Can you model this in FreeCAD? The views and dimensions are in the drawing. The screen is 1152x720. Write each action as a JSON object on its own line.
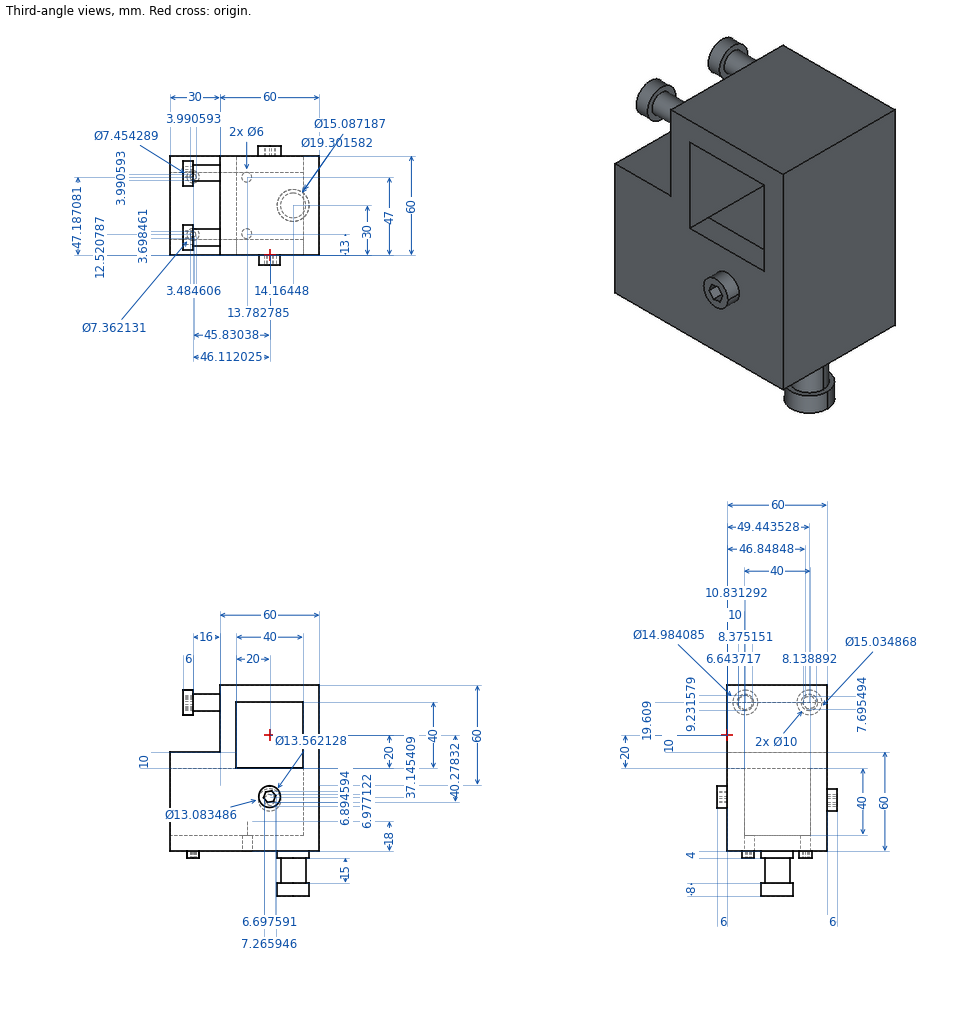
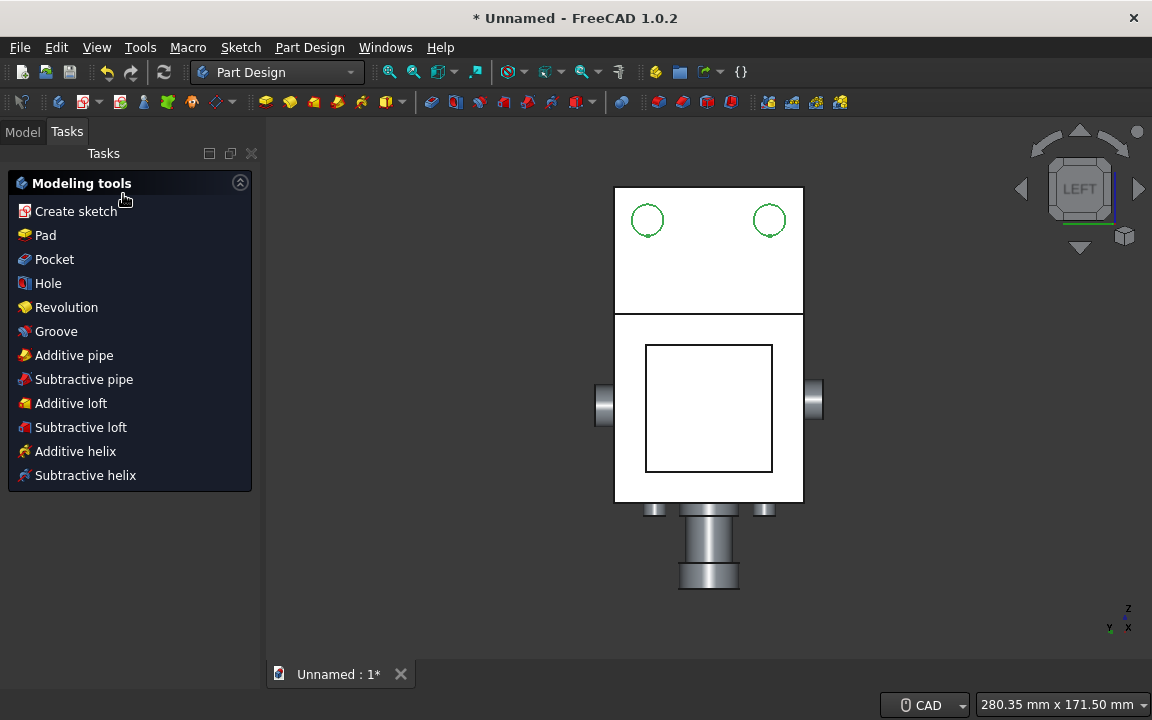
{"action": "left_click", "coordinate": [266, 102]}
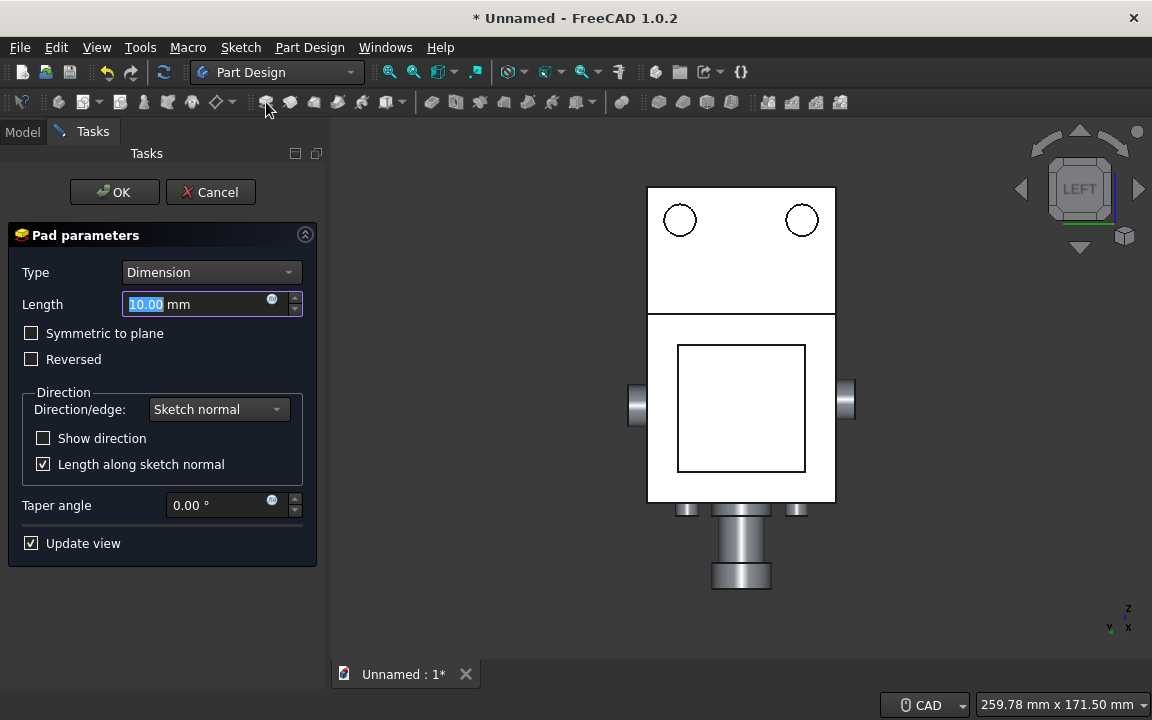
{"action": "type", "text": "16"}
{"action": "key", "text": "Tab"}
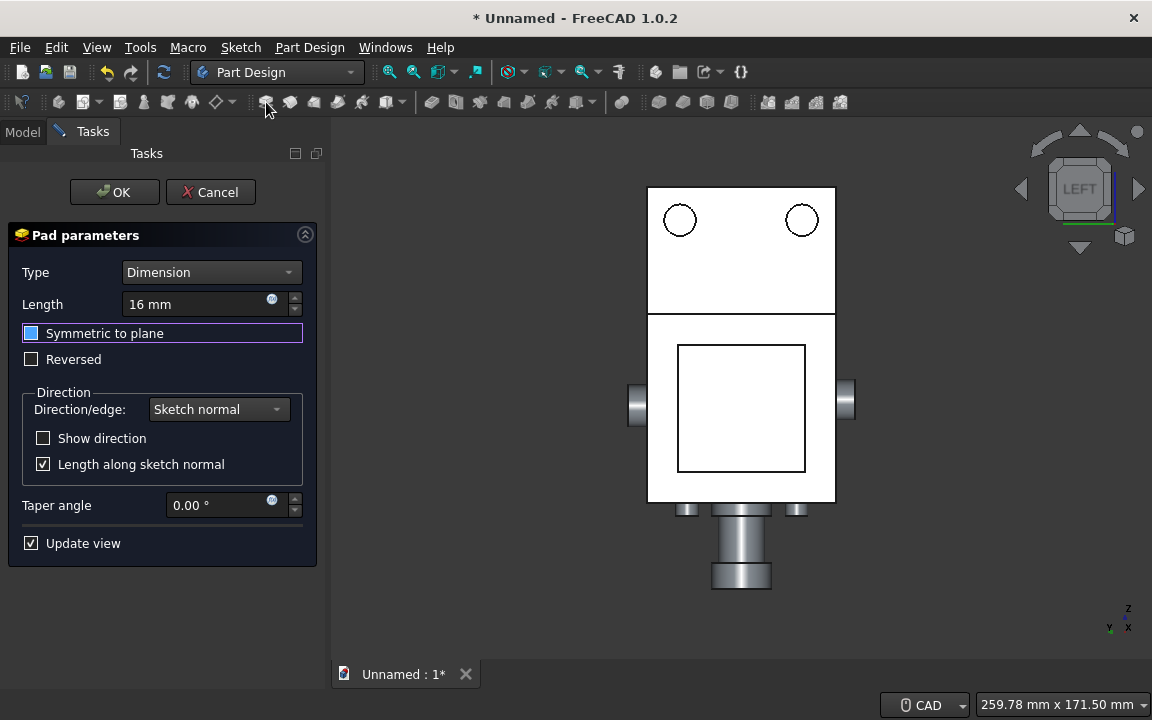
{"action": "left_click", "coordinate": [115, 192]}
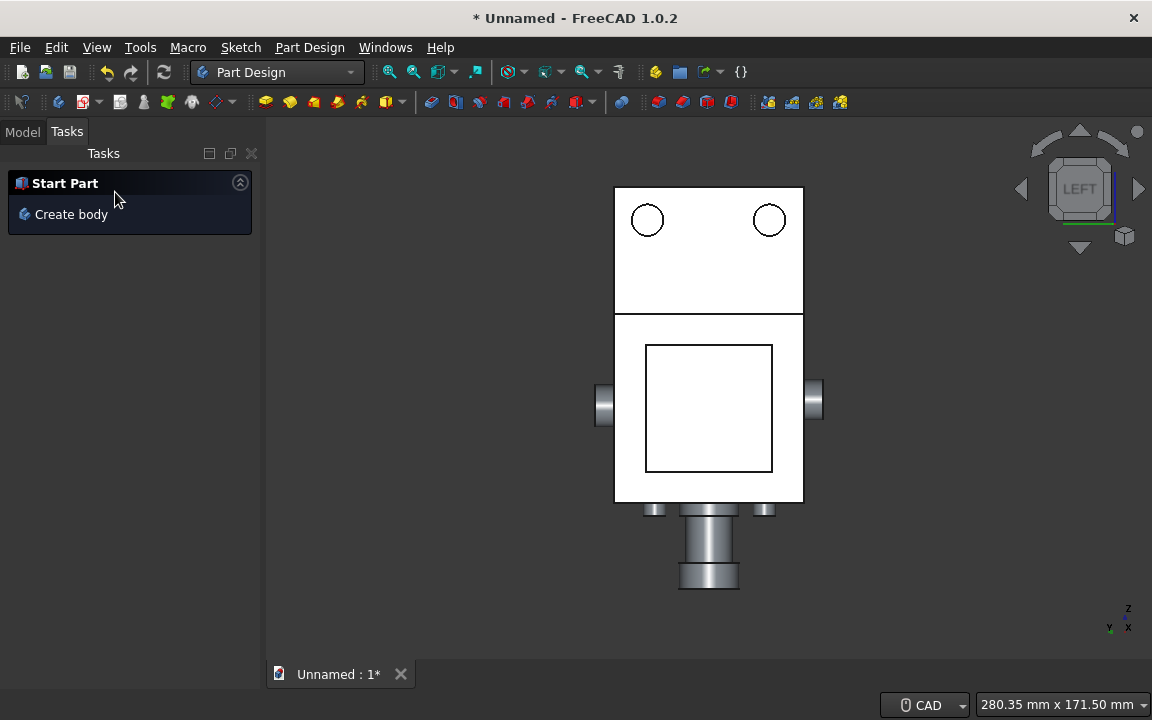
{"action": "left_click", "coordinate": [770, 219]}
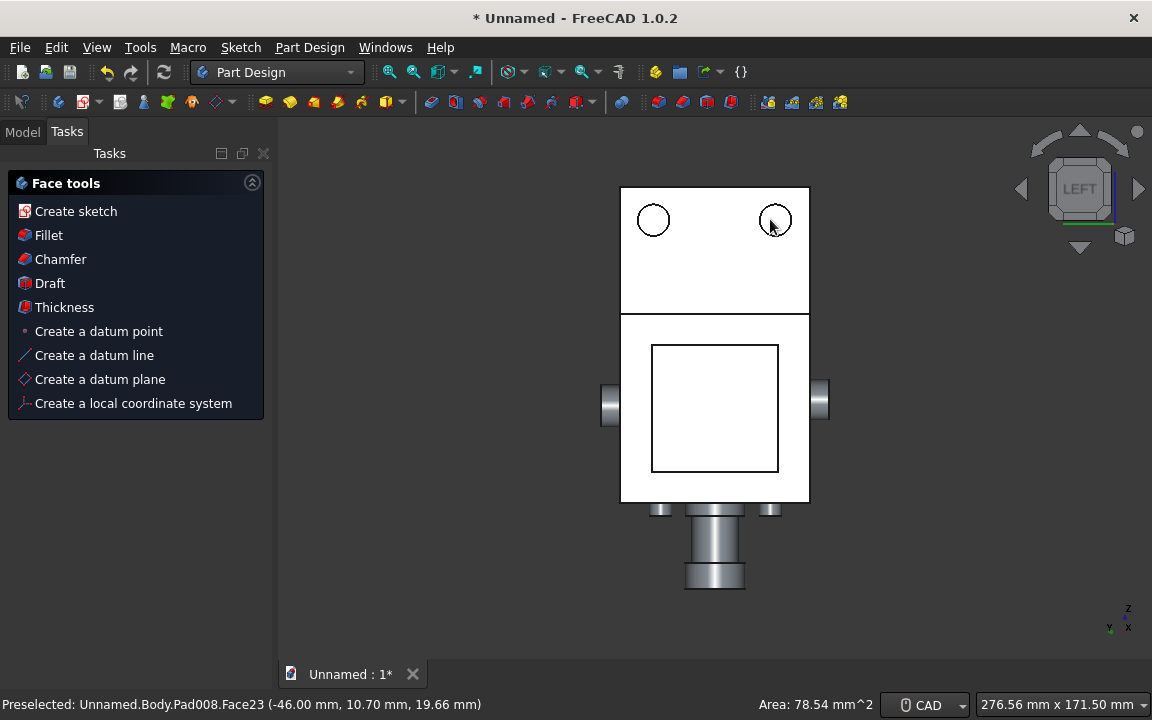
{"action": "left_click", "coordinate": [84, 102]}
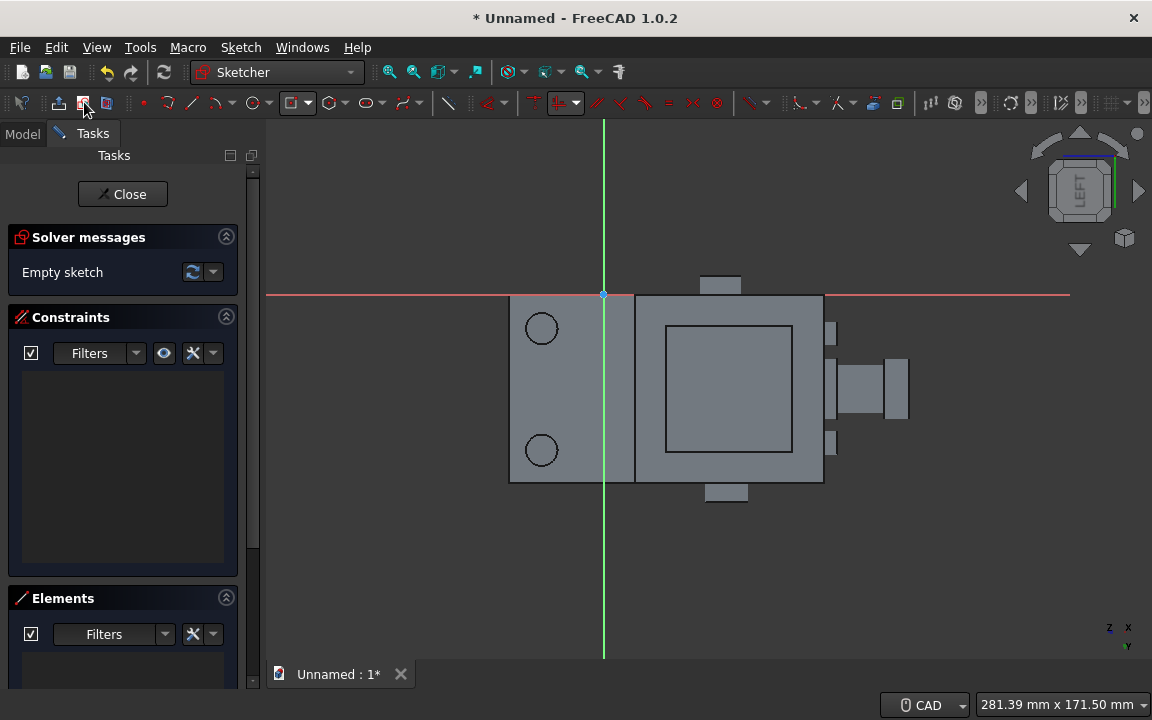
{"action": "scroll", "coordinate": [464, 378], "scroll_direction": "up", "scroll_amount": 3}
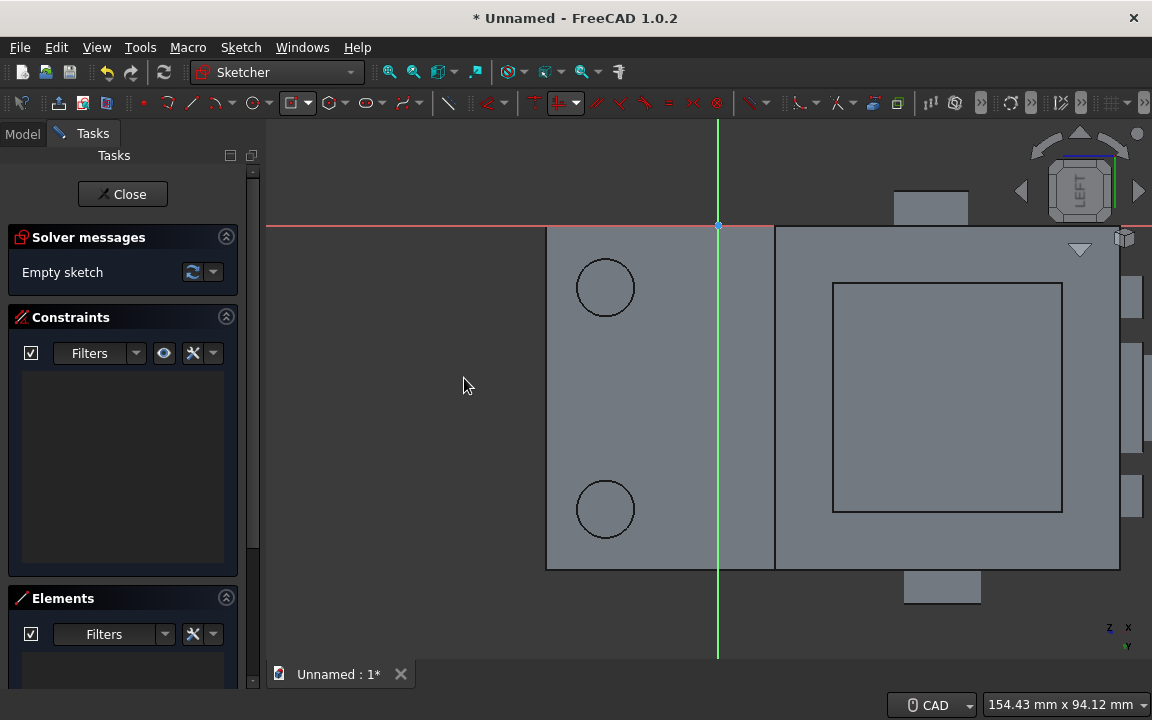
{"action": "left_click", "coordinate": [330, 104]}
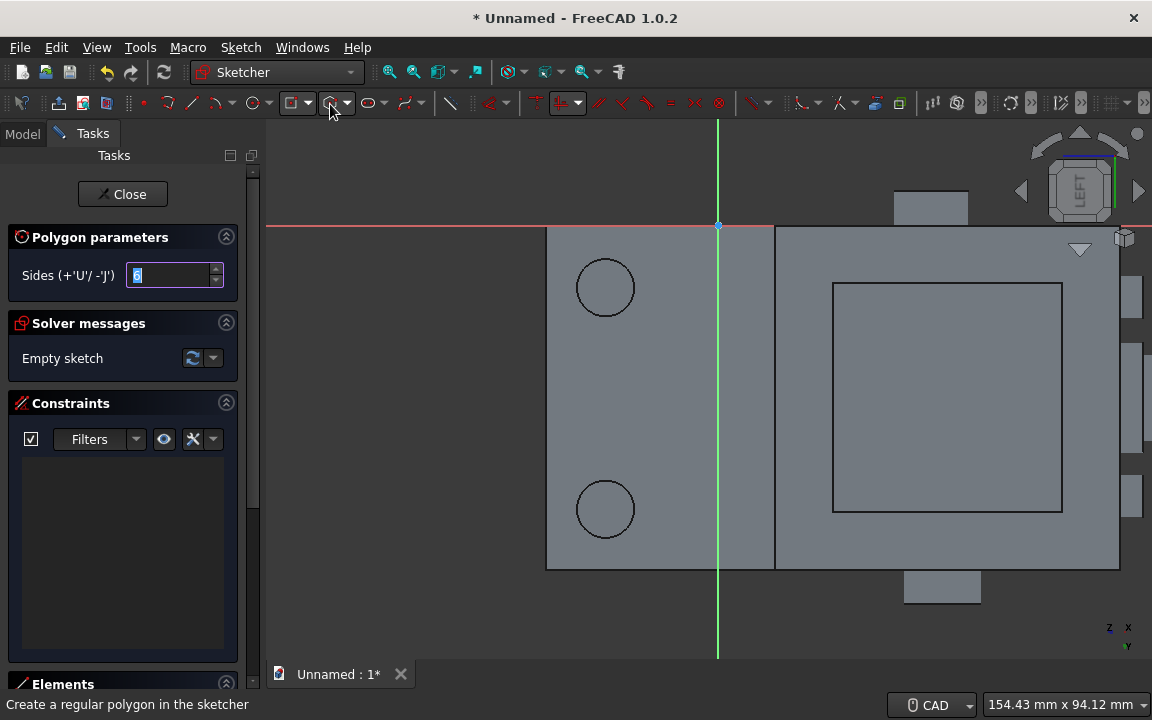
{"action": "left_click", "coordinate": [606, 288]}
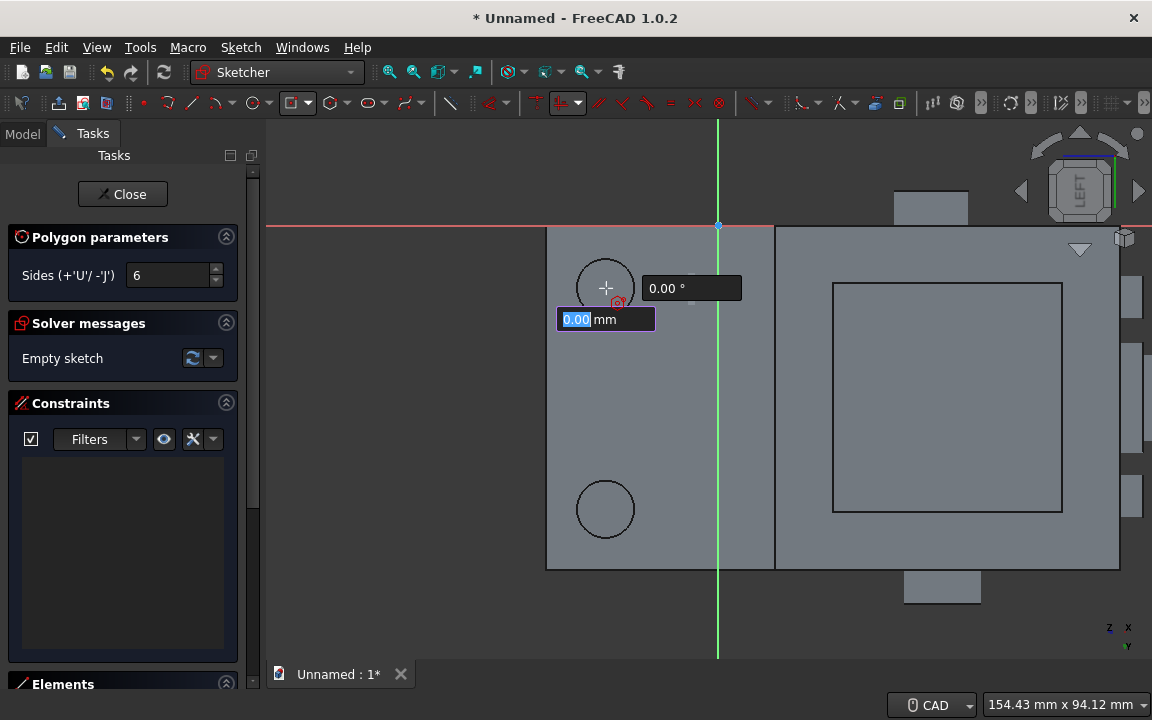
{"action": "left_click", "coordinate": [594, 312]}
{"action": "right_click", "coordinate": [594, 312]}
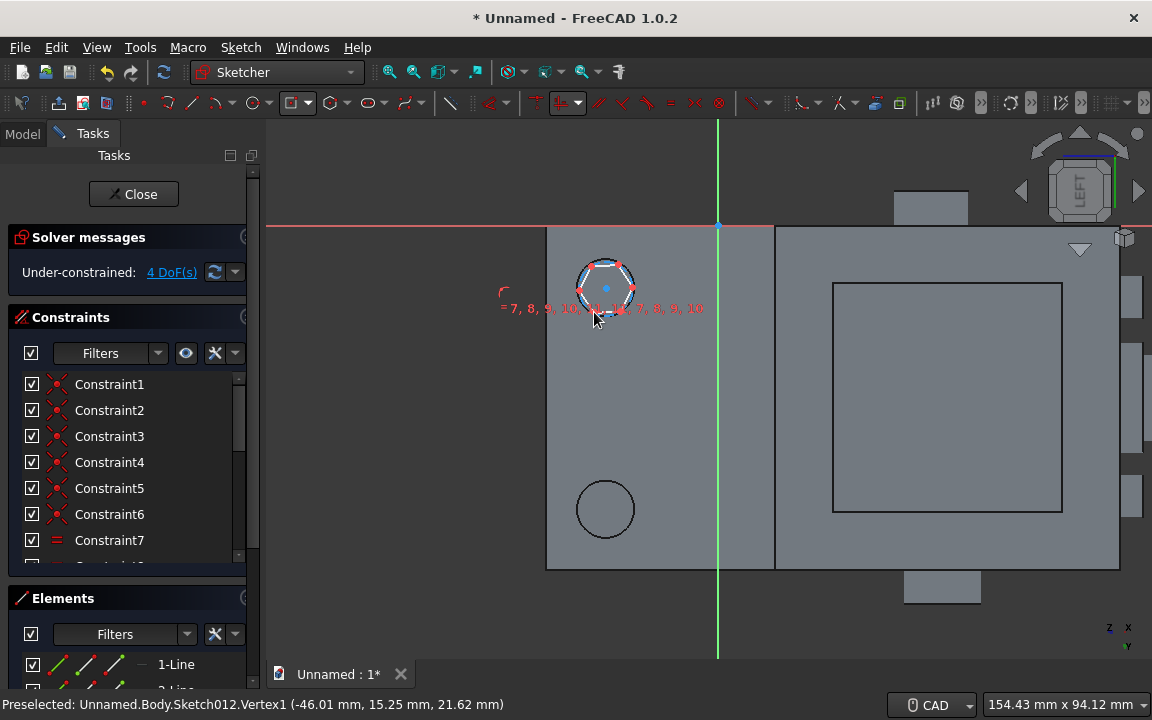
{"action": "left_click", "coordinate": [330, 104]}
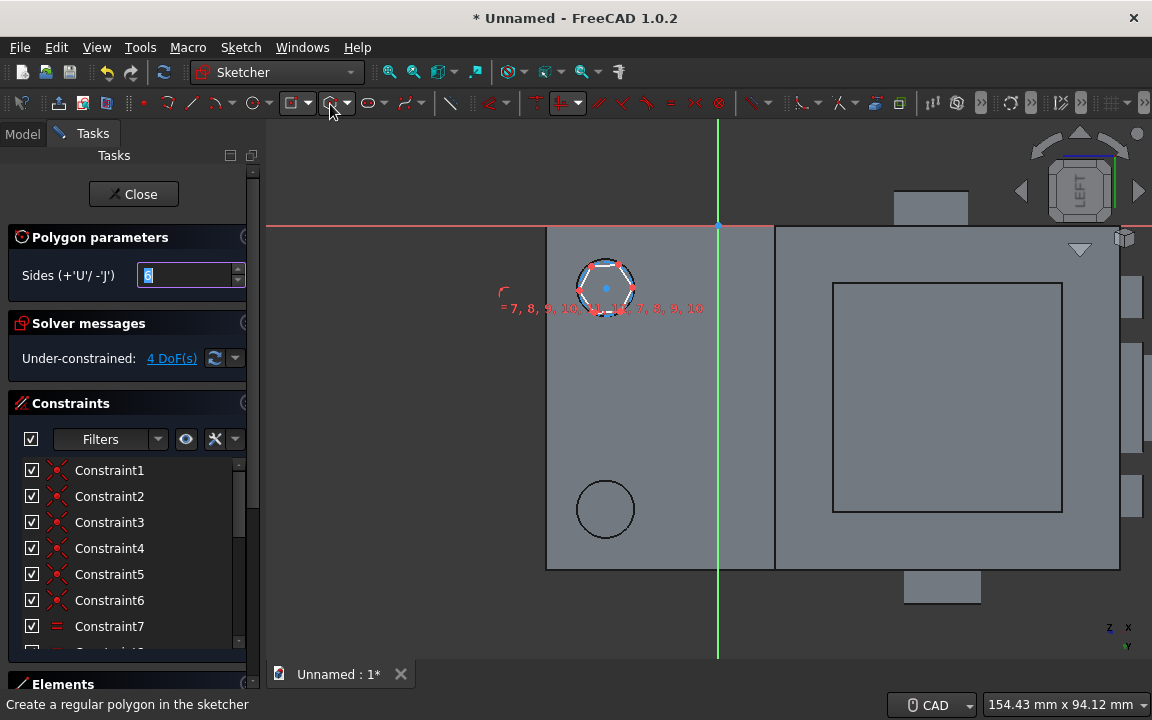
{"action": "scroll", "coordinate": [606, 509], "scroll_direction": "up", "scroll_amount": 2}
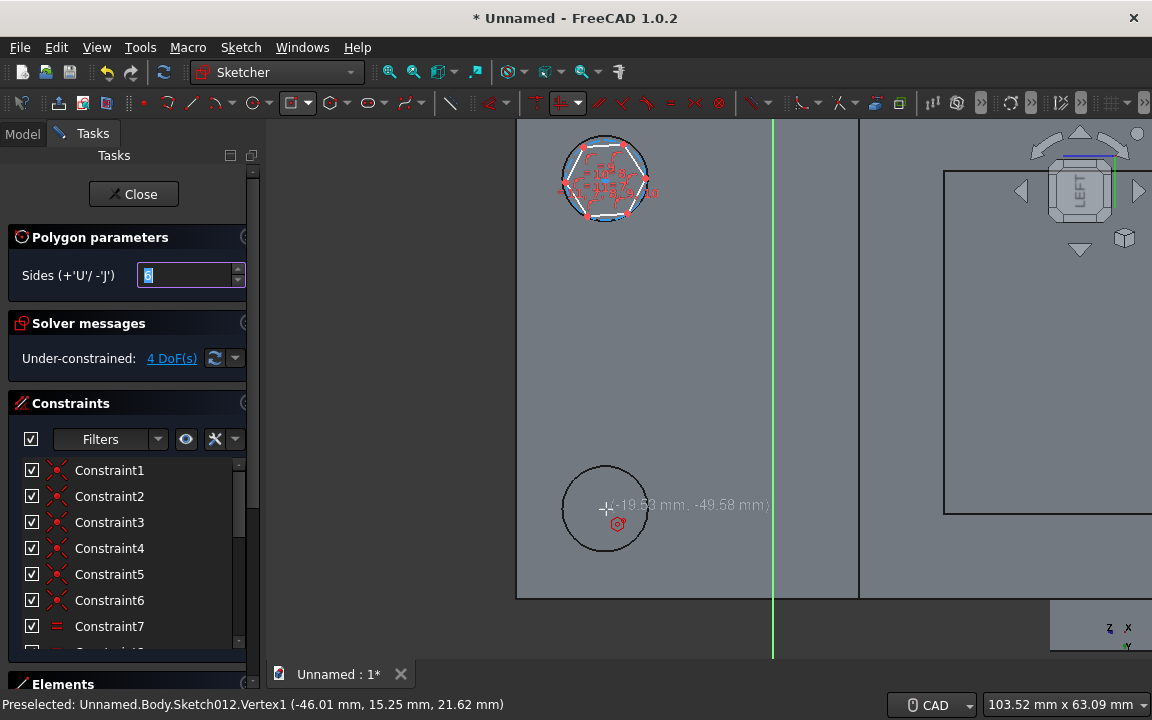
{"action": "left_click", "coordinate": [605, 509]}